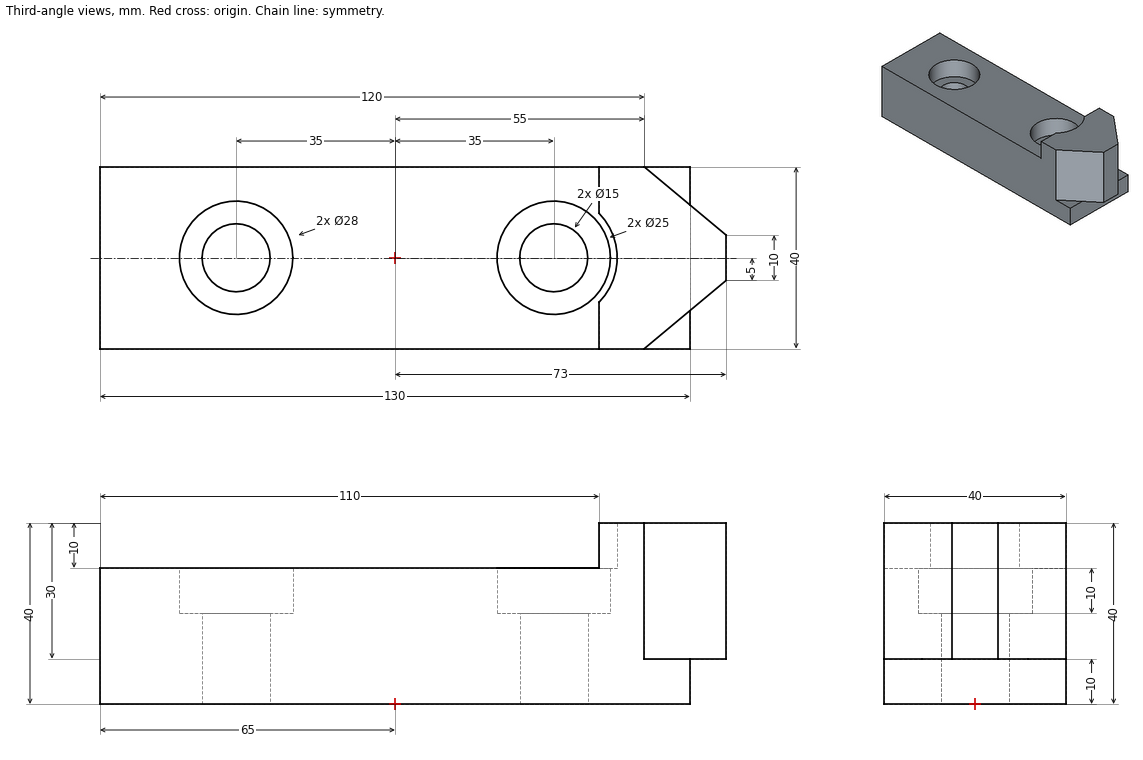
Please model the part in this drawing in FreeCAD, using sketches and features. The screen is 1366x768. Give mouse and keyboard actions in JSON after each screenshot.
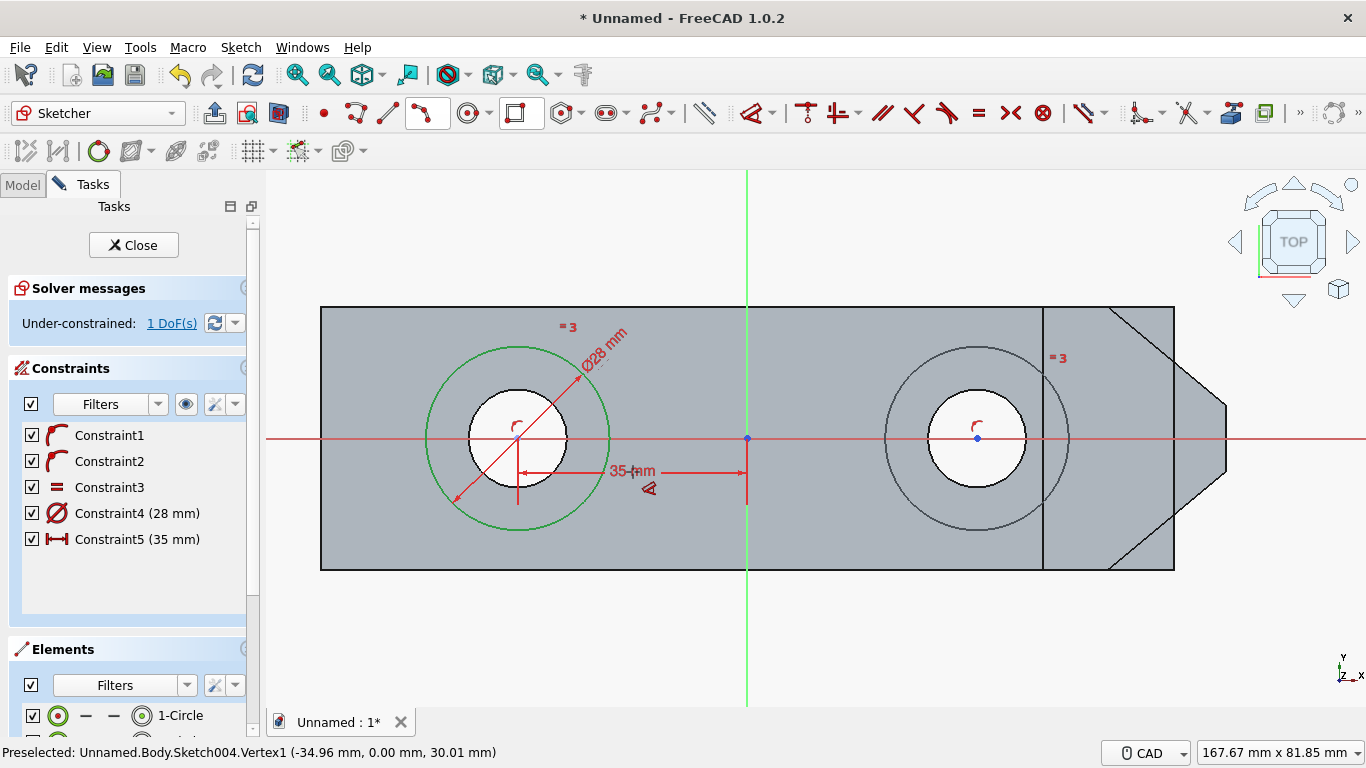
{"action": "left_click", "coordinate": [977, 438]}
{"action": "left_click", "coordinate": [862, 472]}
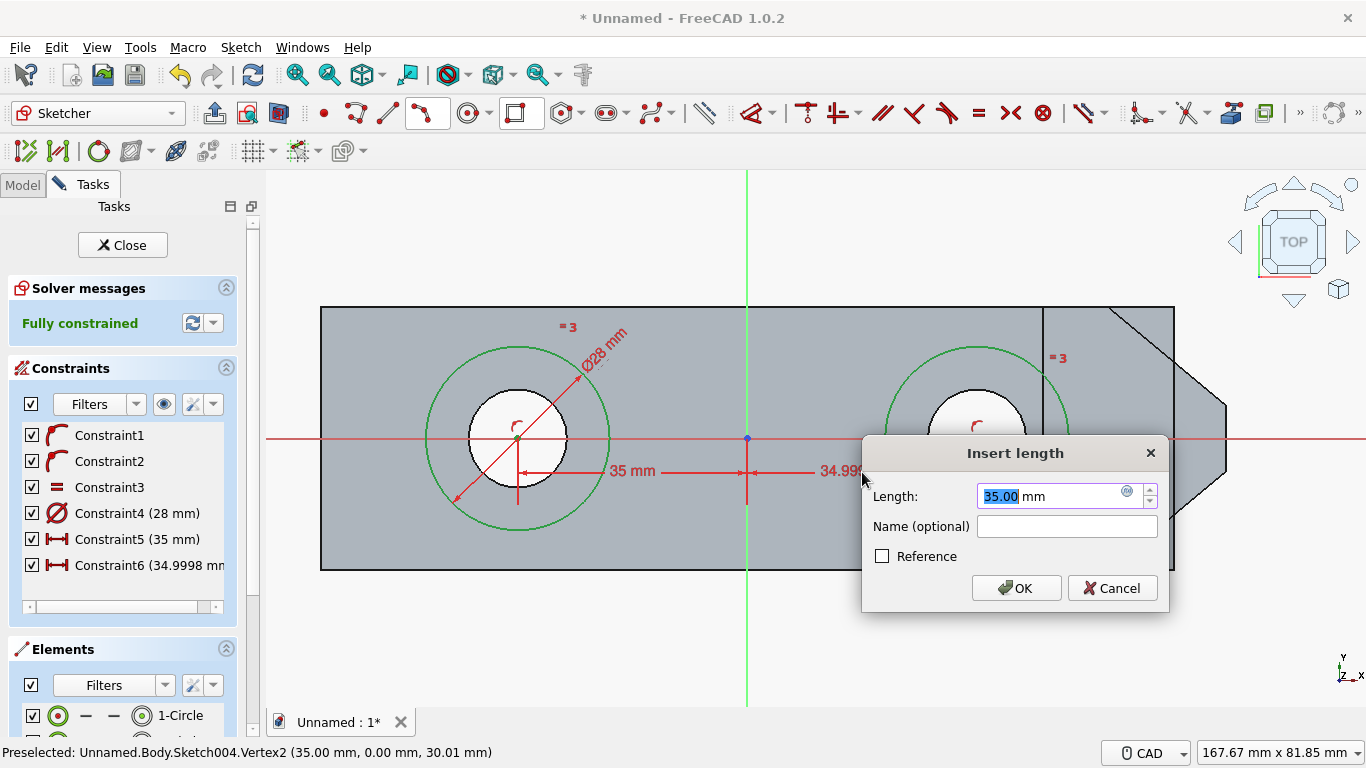
{"action": "type", "text": "35"}
{"action": "key", "text": "Return"}
{"action": "key", "text": "Escape"}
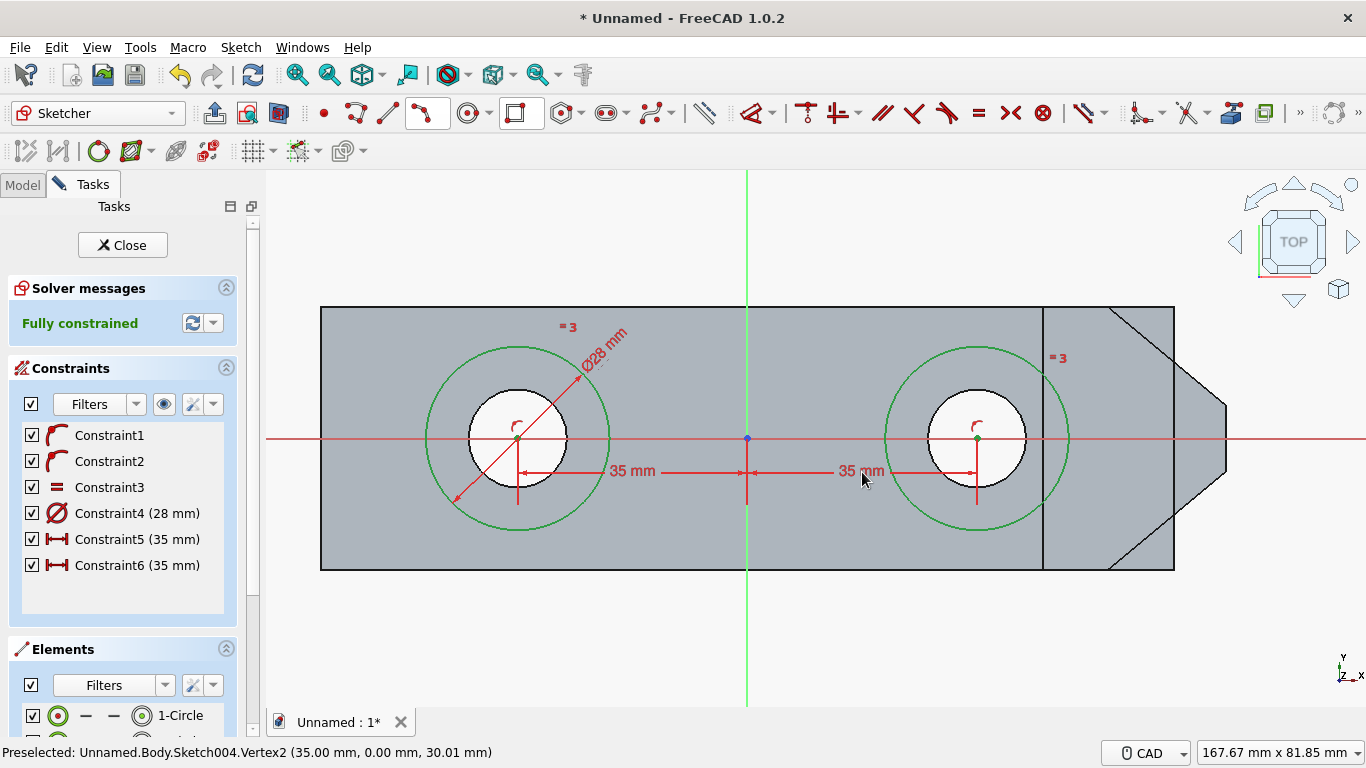
{"action": "left_click", "coordinate": [123, 245]}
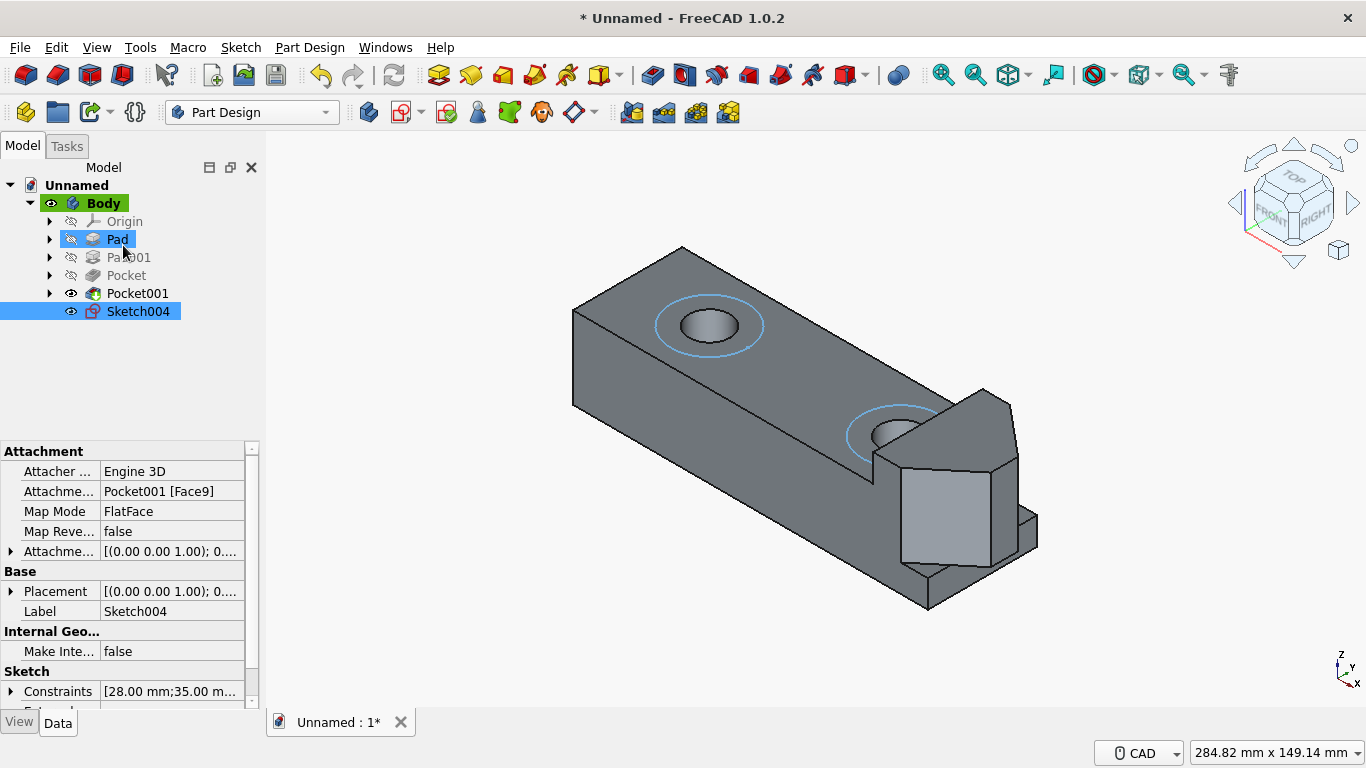
{"action": "left_click", "coordinate": [654, 76]}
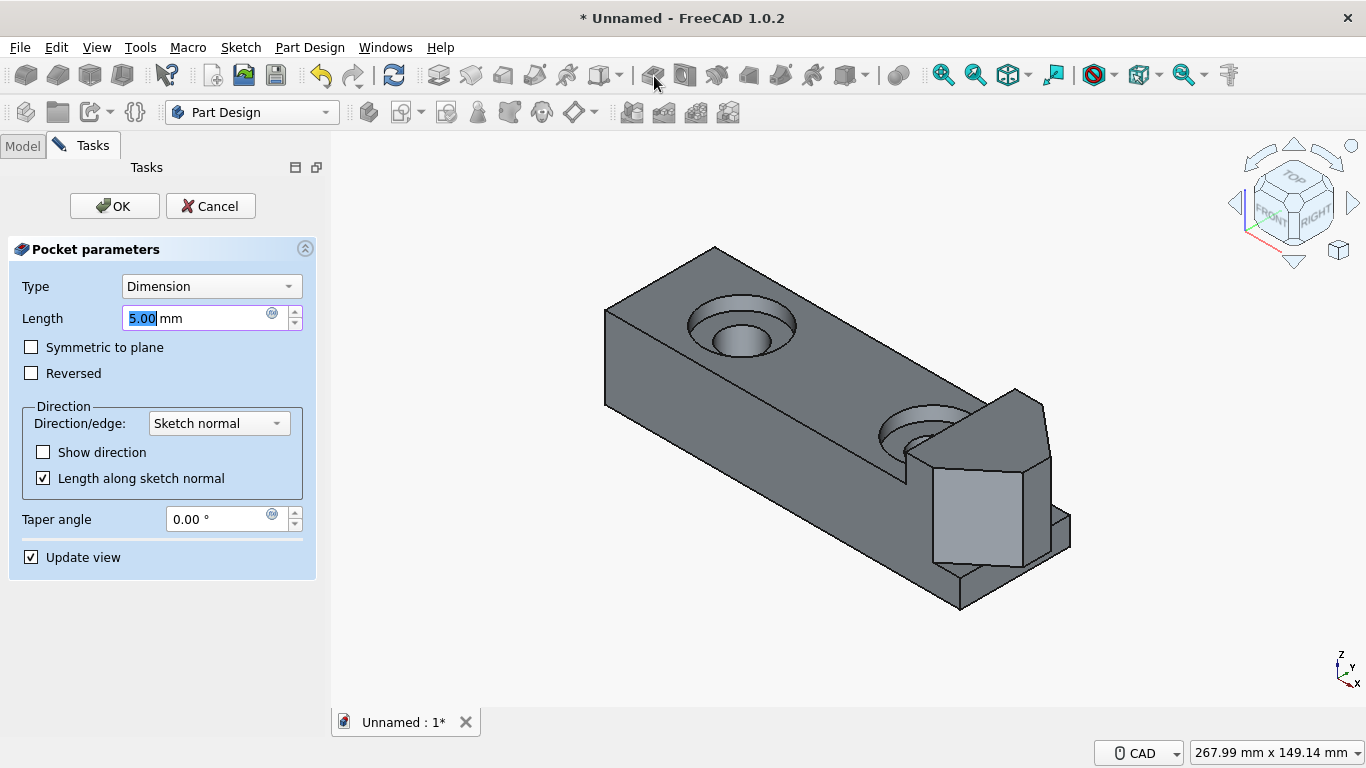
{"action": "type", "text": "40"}
{"action": "key", "text": "Tab"}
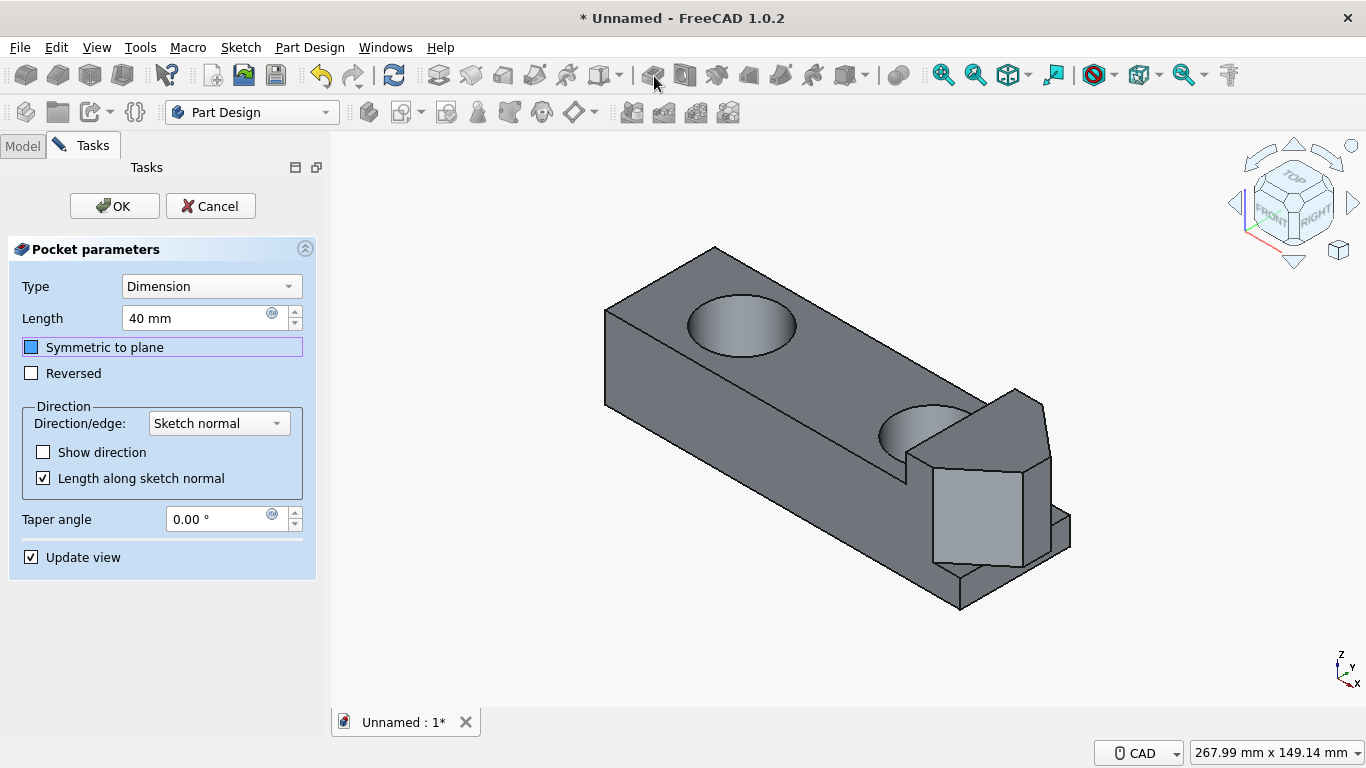
{"action": "left_click", "coordinate": [30, 373]}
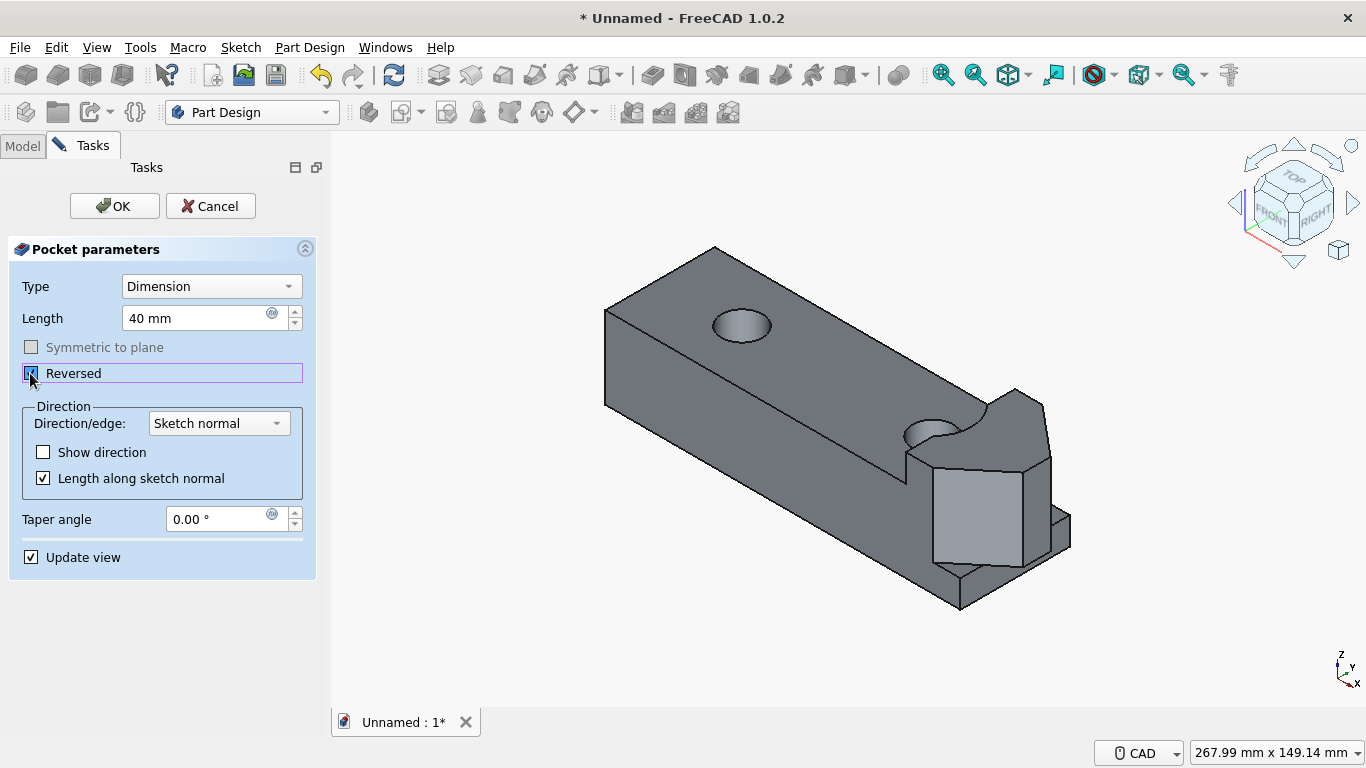
{"action": "left_click", "coordinate": [115, 206]}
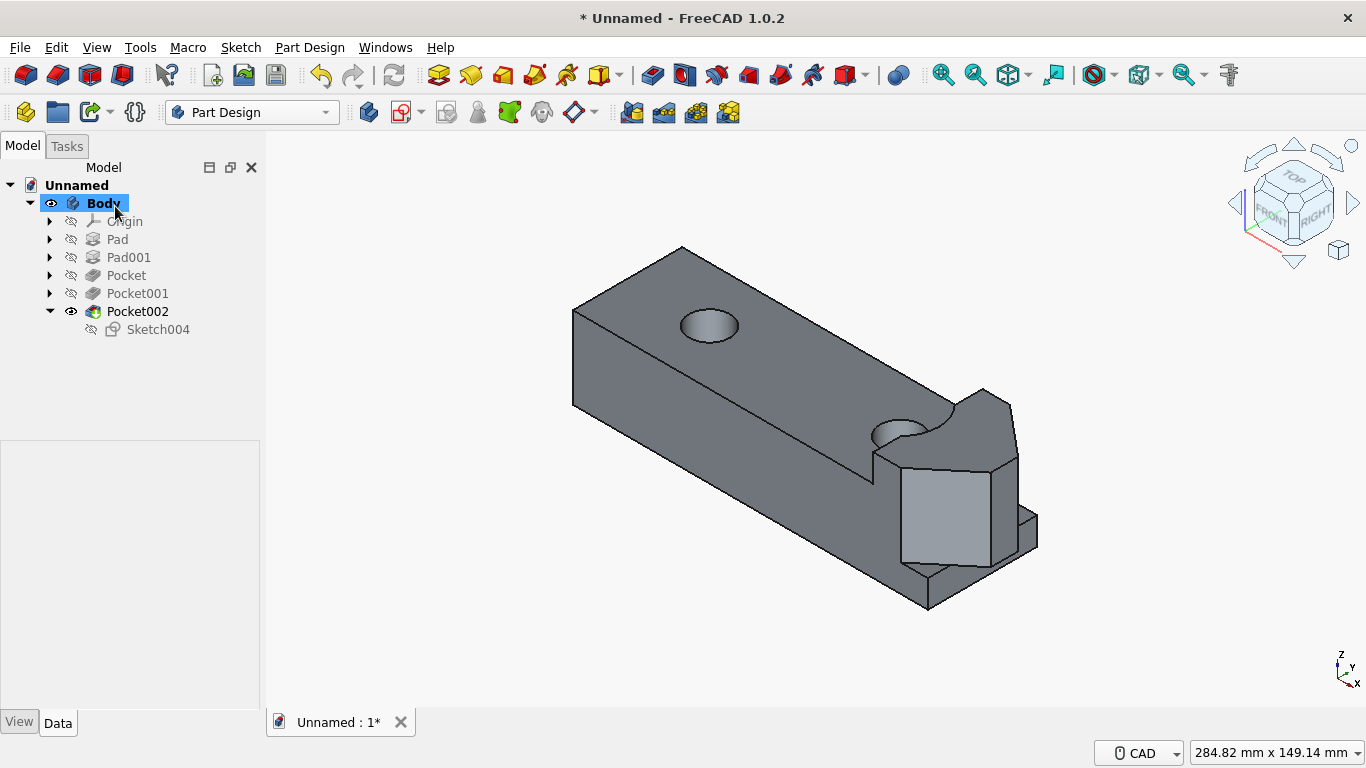
{"action": "left_click", "coordinate": [783, 368]}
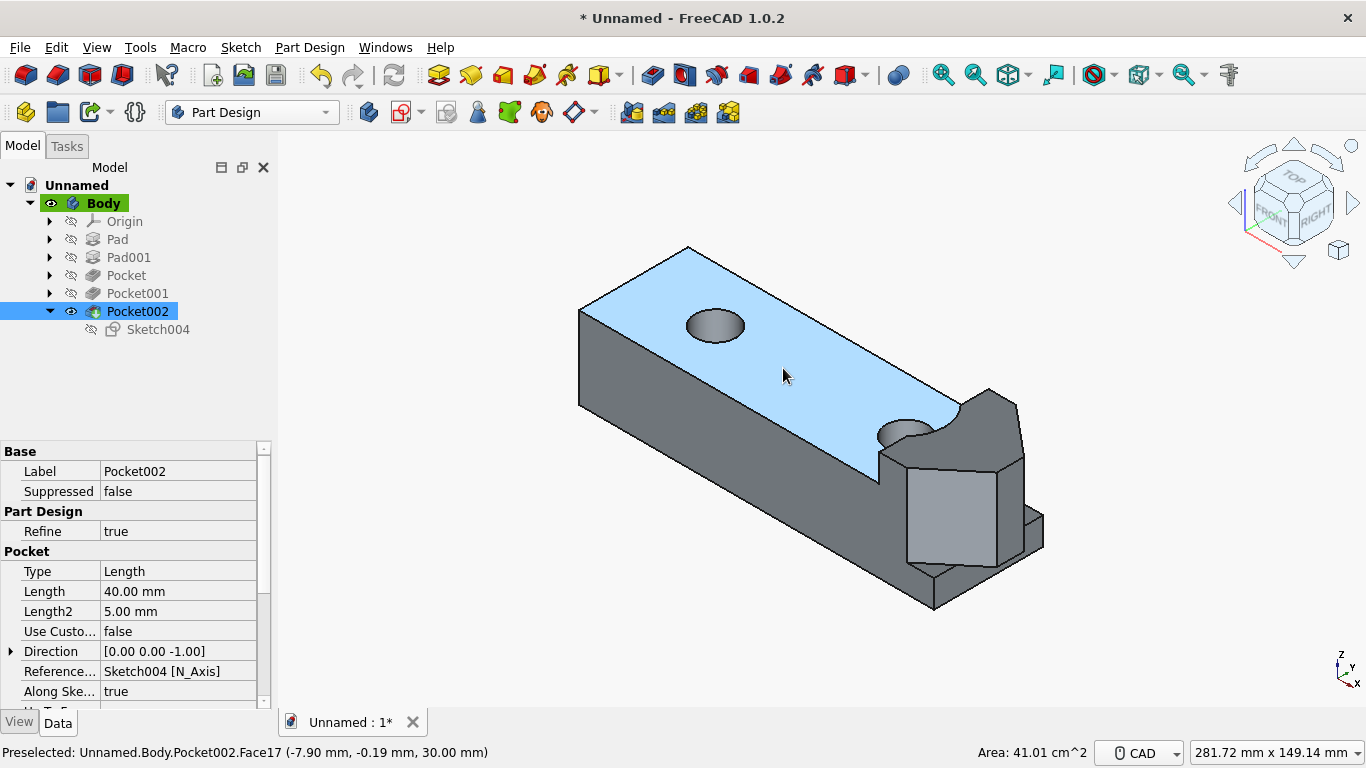
{"action": "left_click", "coordinate": [402, 112]}